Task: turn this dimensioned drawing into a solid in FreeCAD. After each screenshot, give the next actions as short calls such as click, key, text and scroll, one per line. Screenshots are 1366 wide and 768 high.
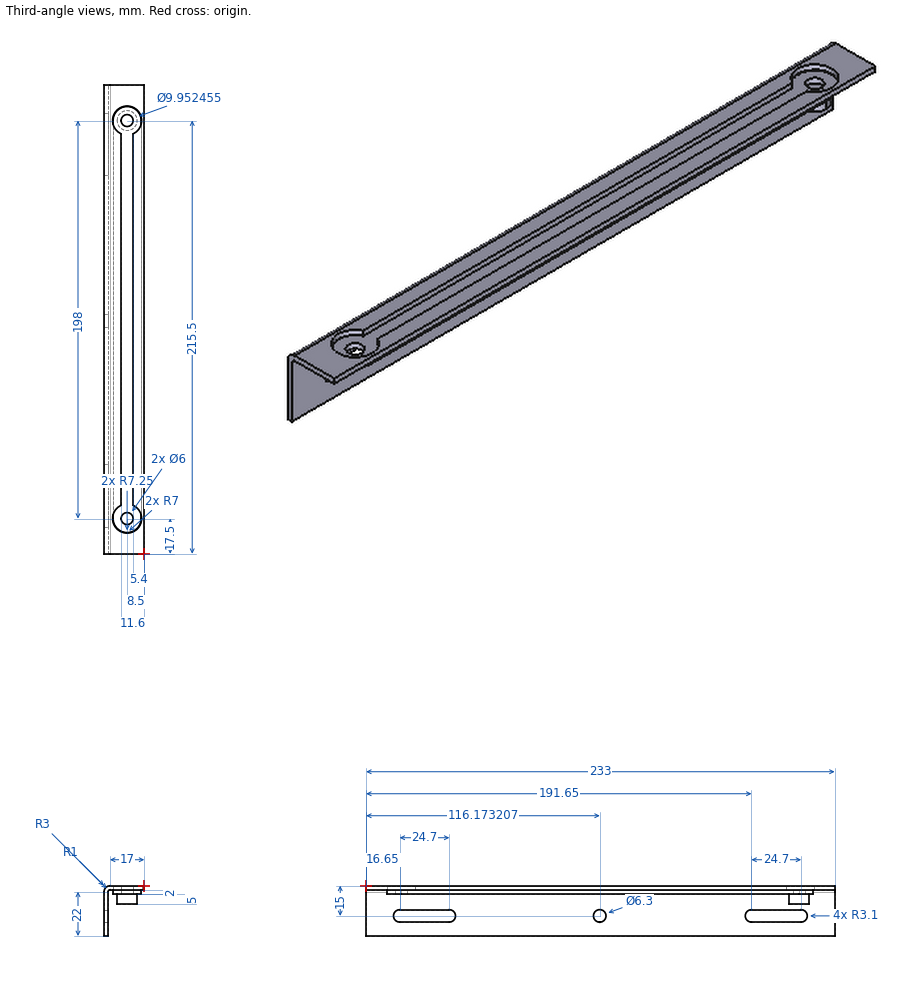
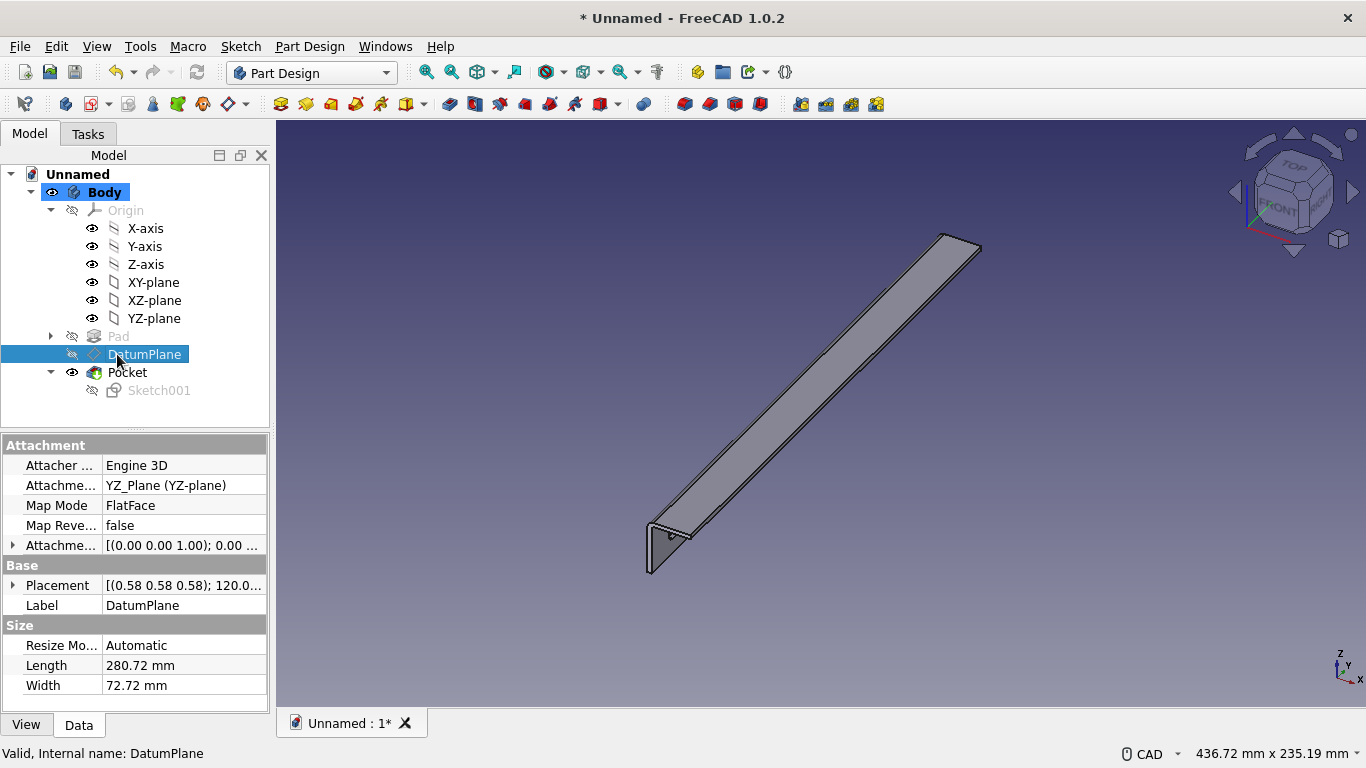
key(5)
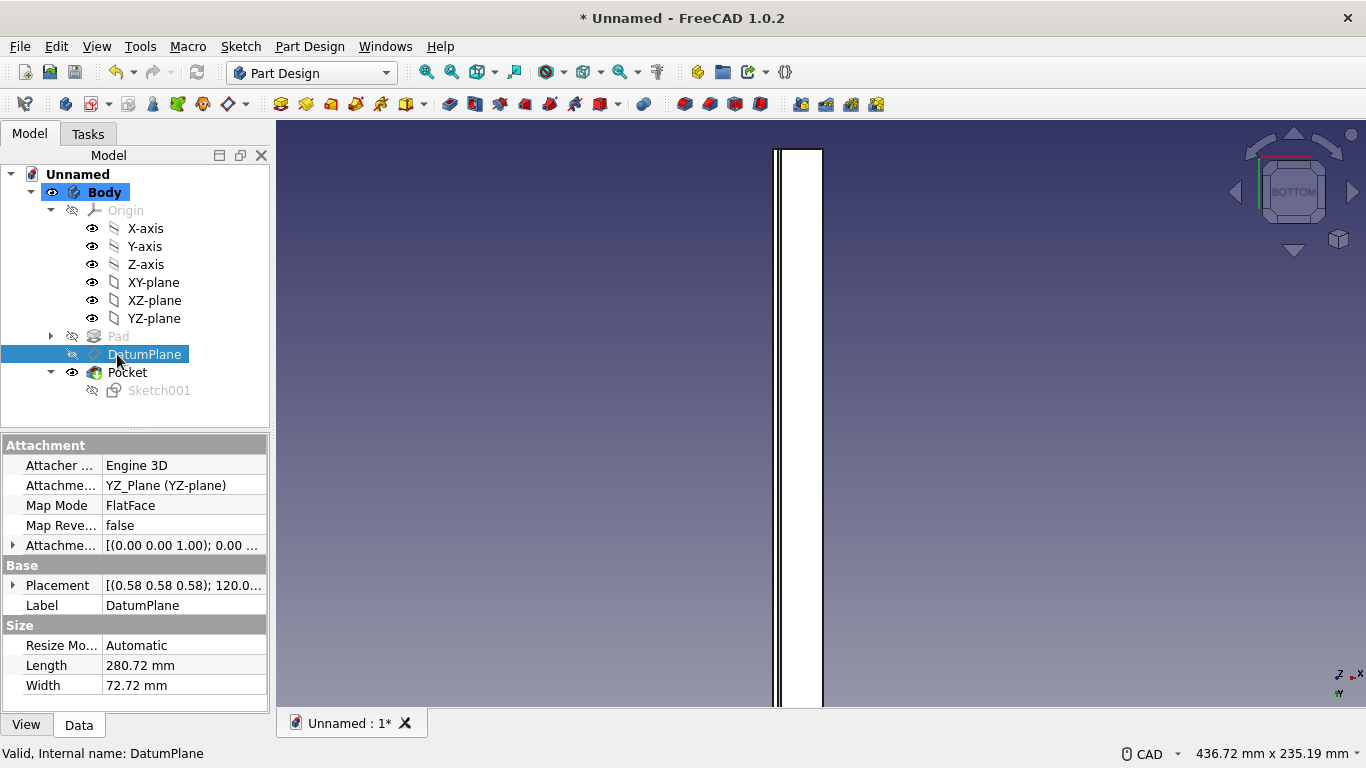
click(427, 72)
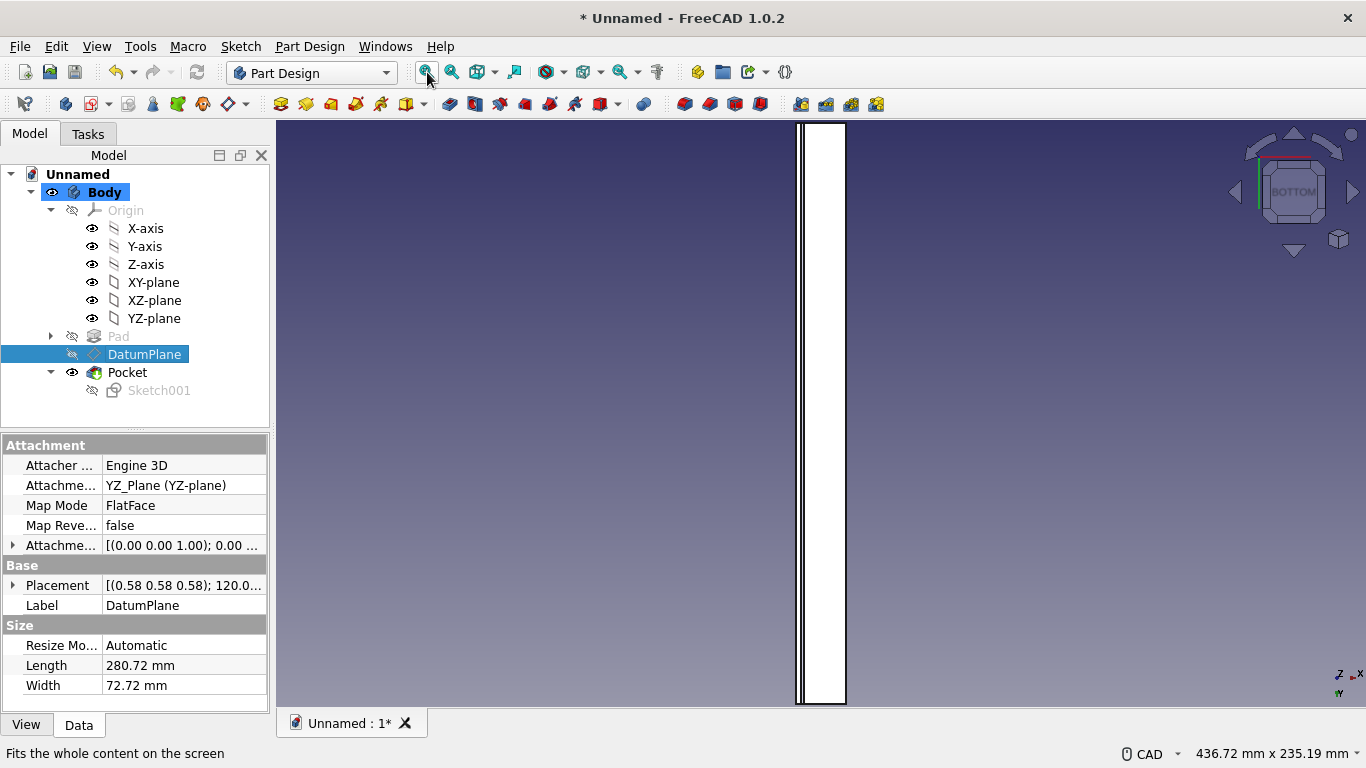
click(825, 662)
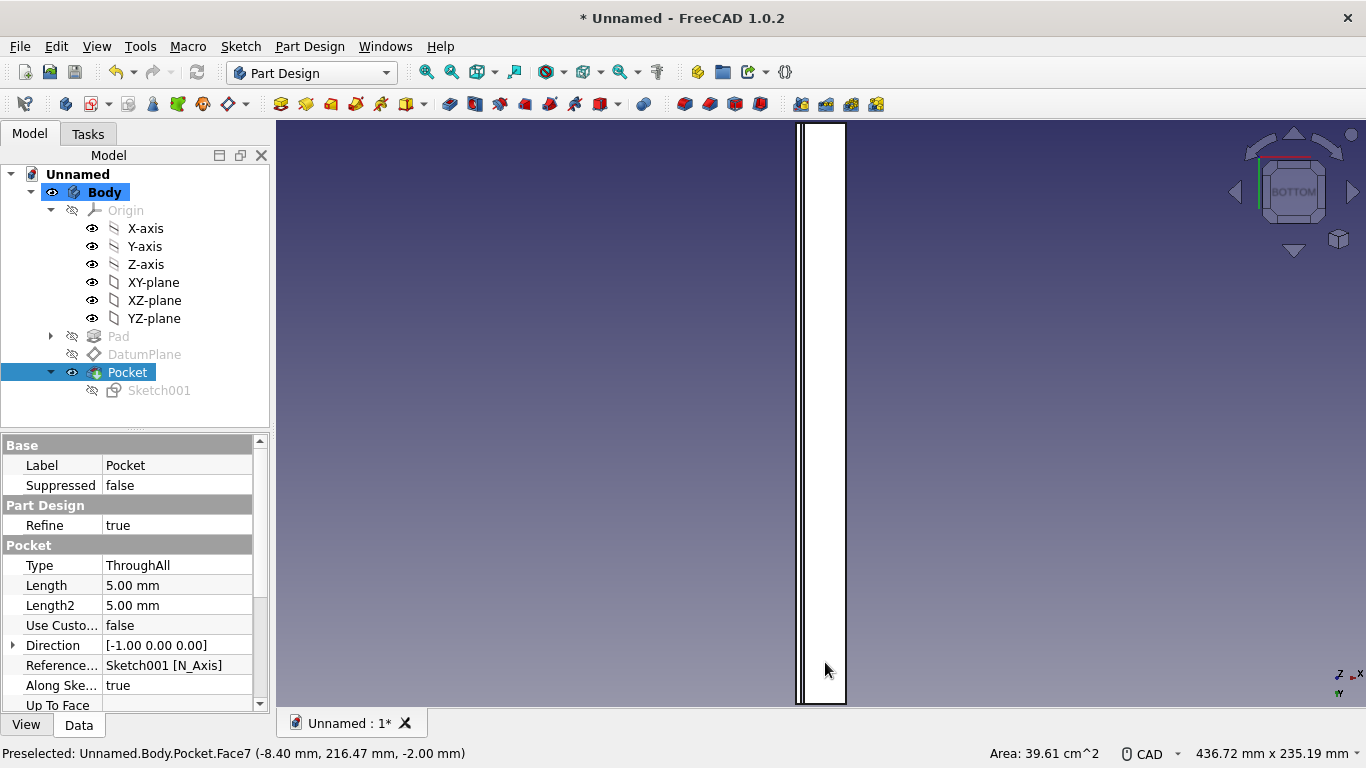
click(90, 104)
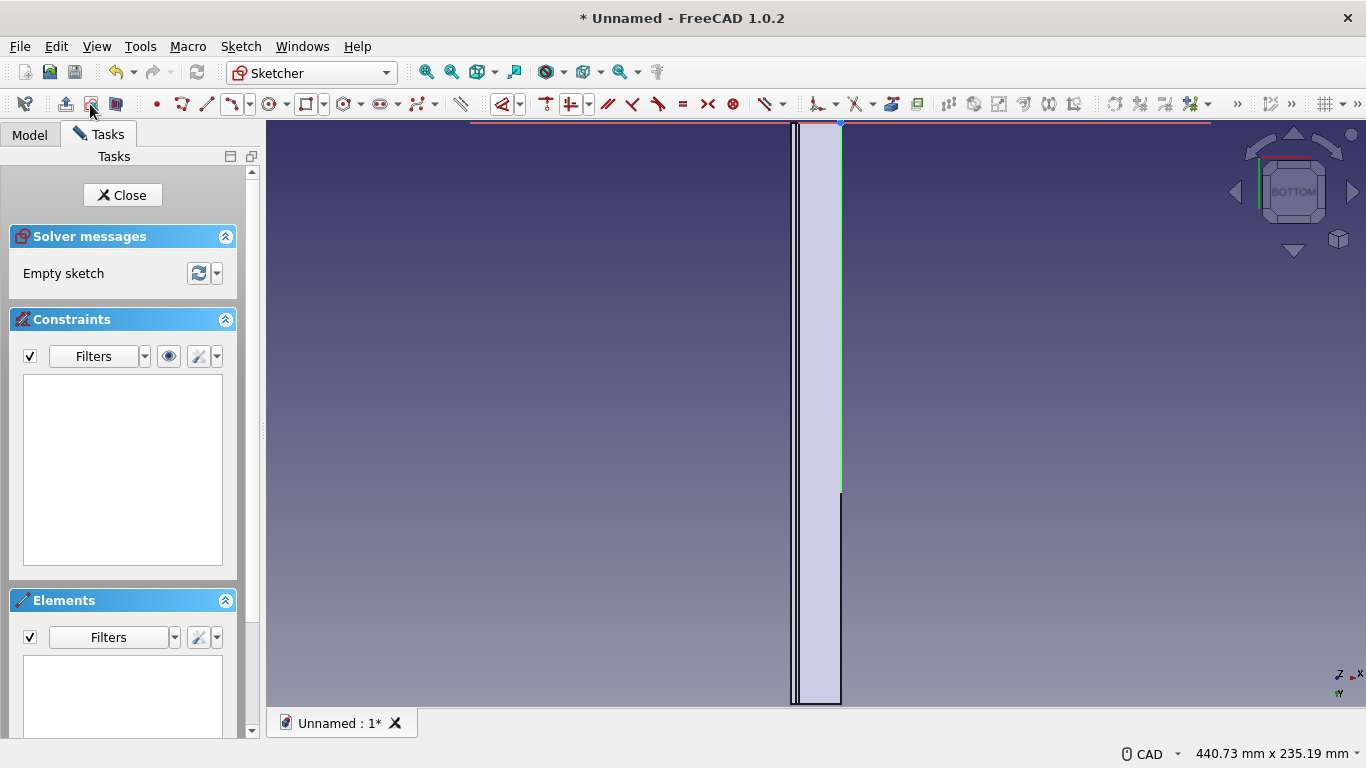
click(116, 104)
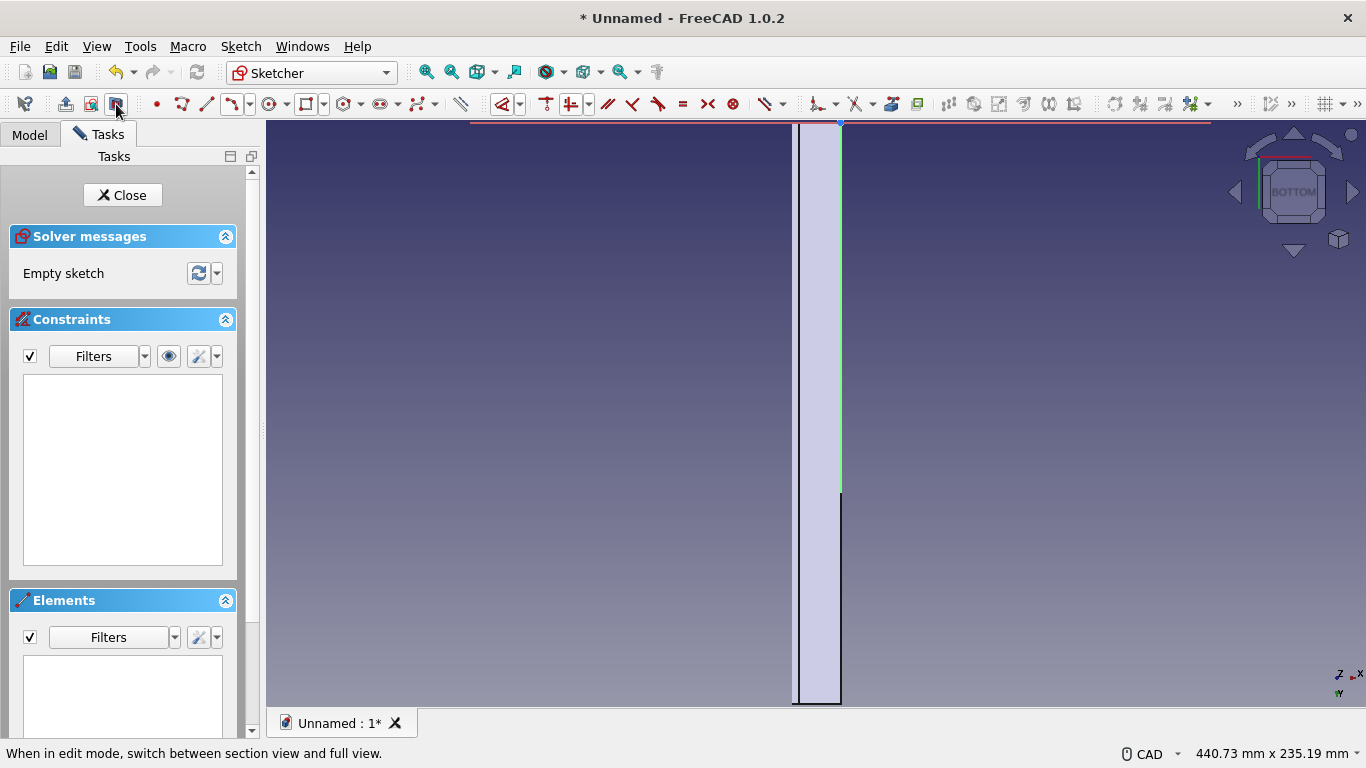
scroll(587, 440, down, 2)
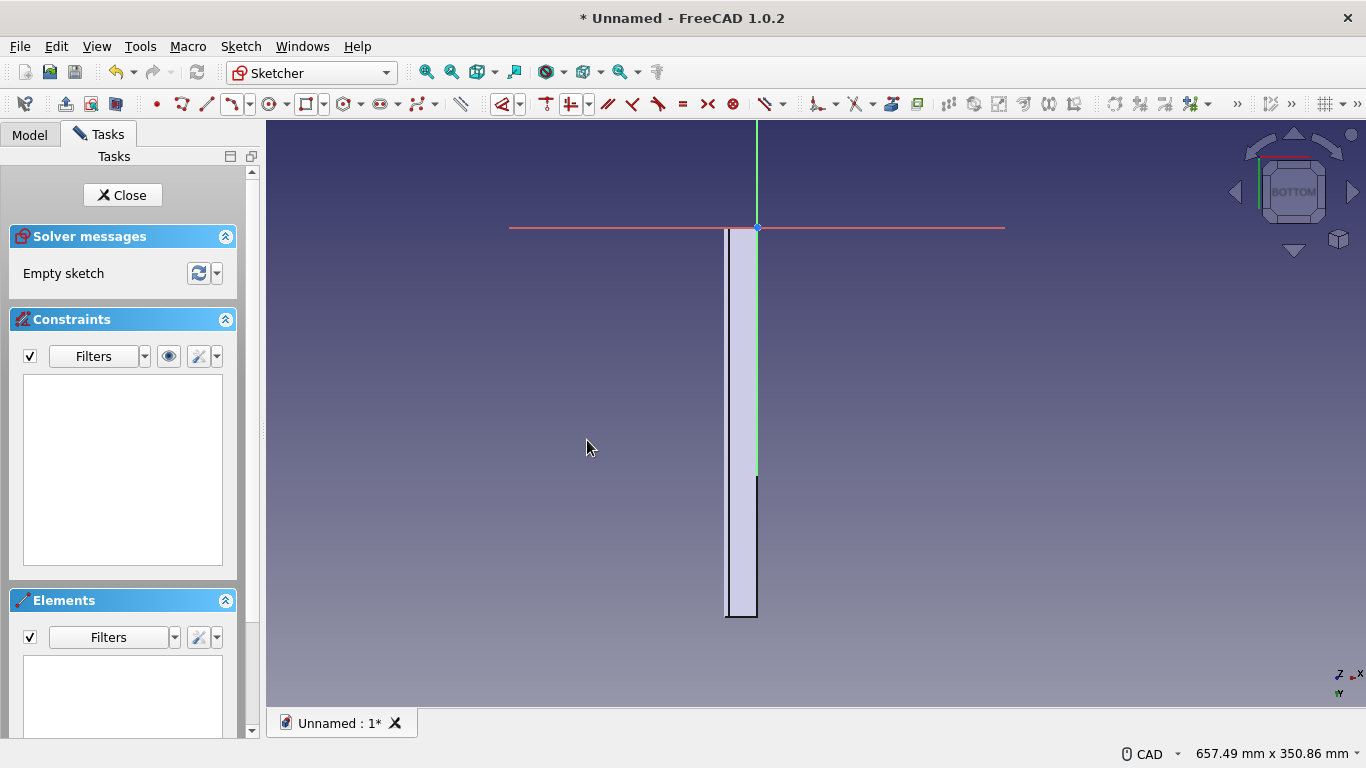
click(207, 104)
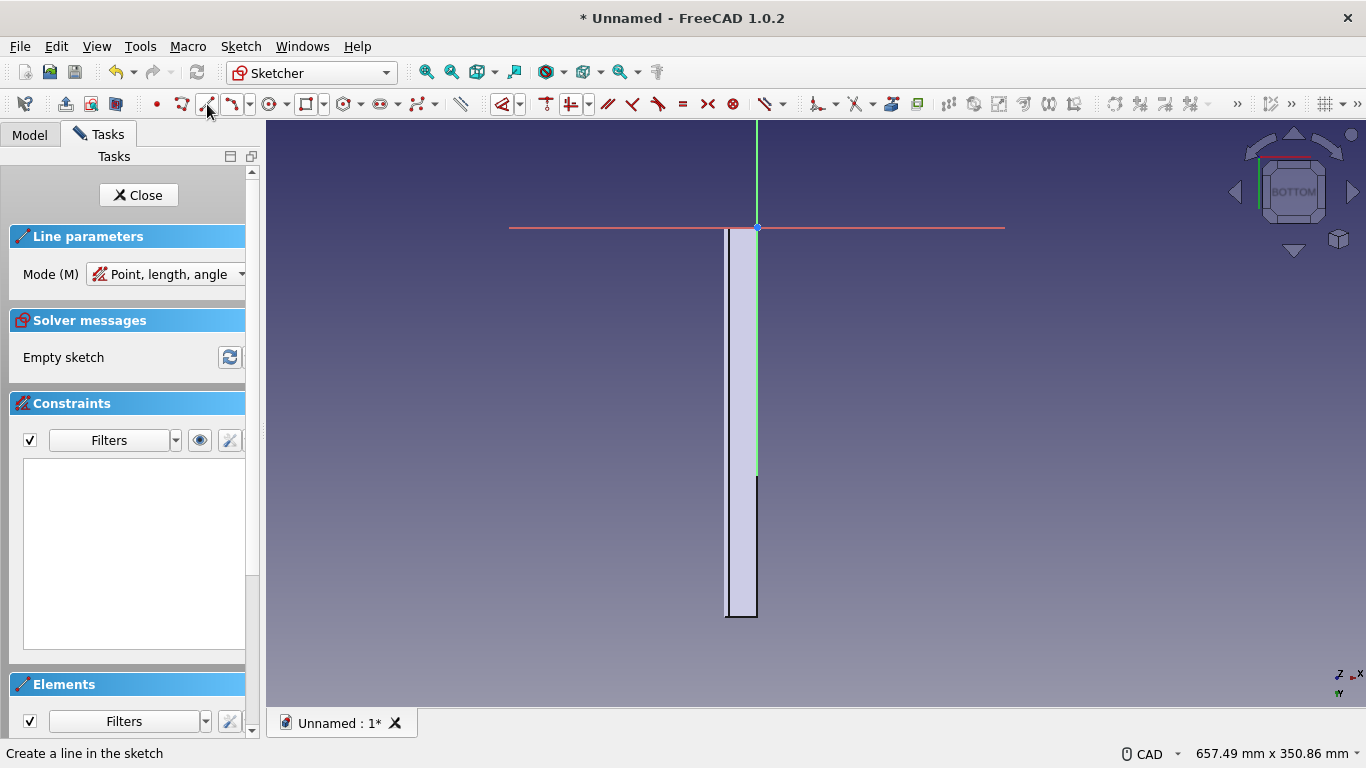
scroll(748, 577, up, 3)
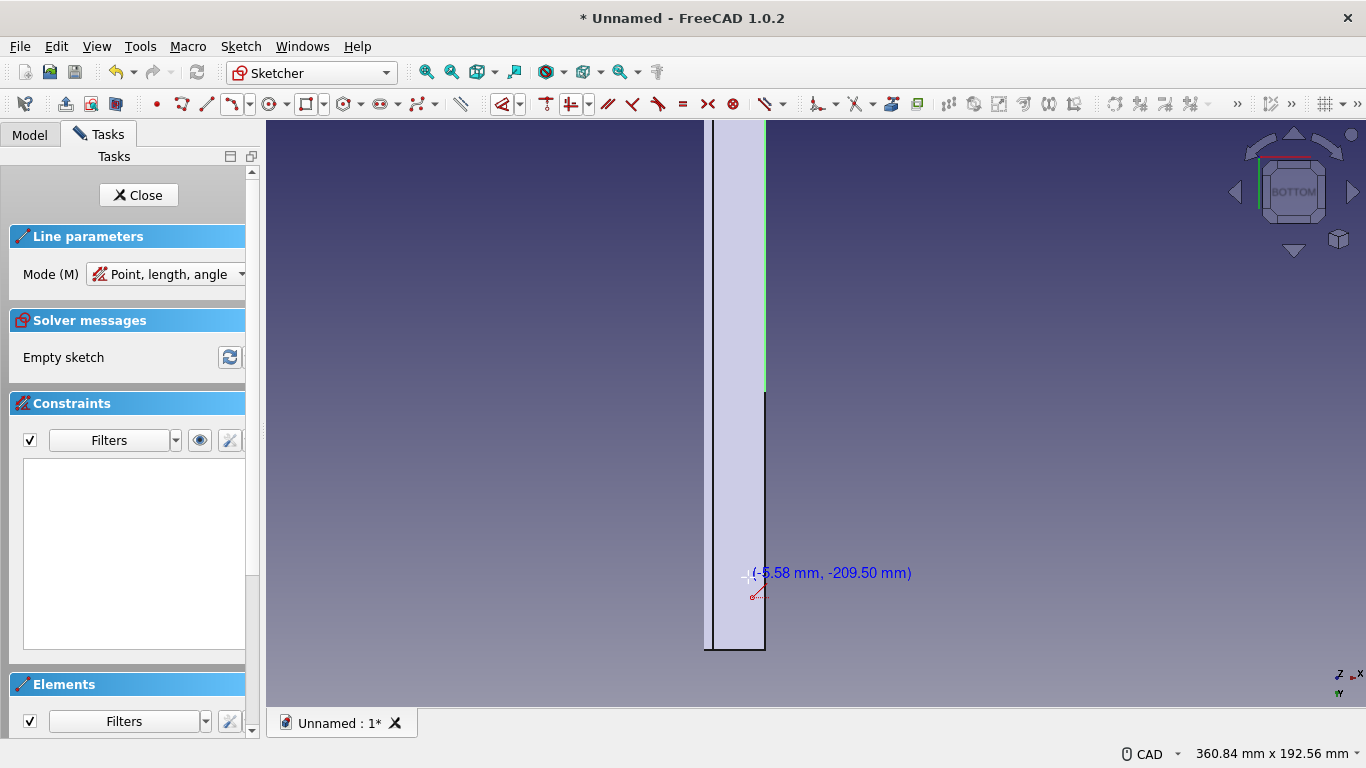
click(748, 577)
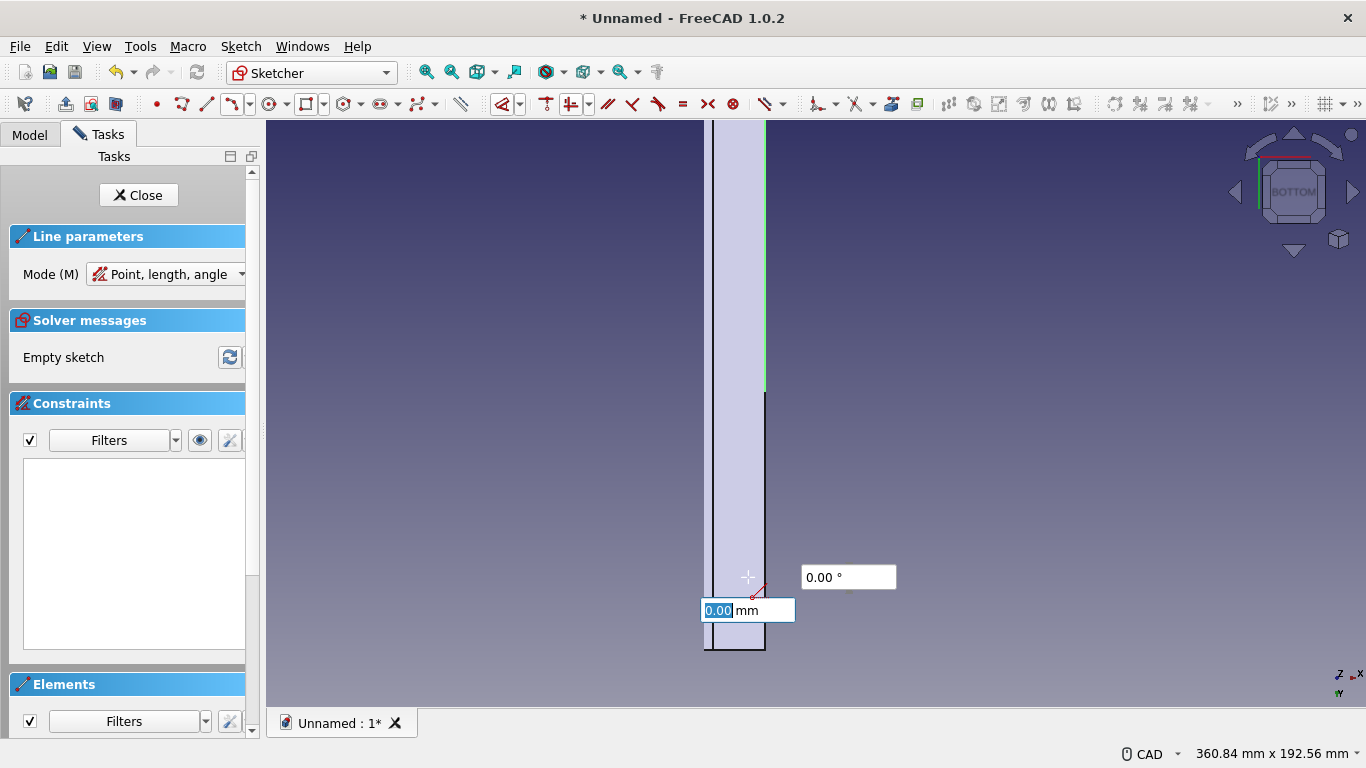
scroll(748, 577, down, 3)